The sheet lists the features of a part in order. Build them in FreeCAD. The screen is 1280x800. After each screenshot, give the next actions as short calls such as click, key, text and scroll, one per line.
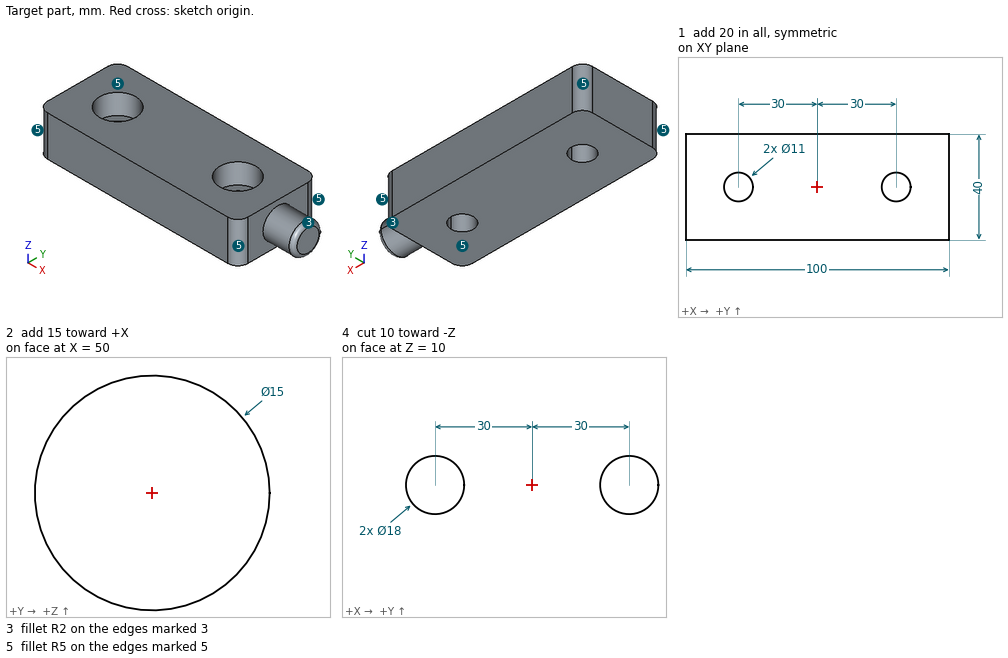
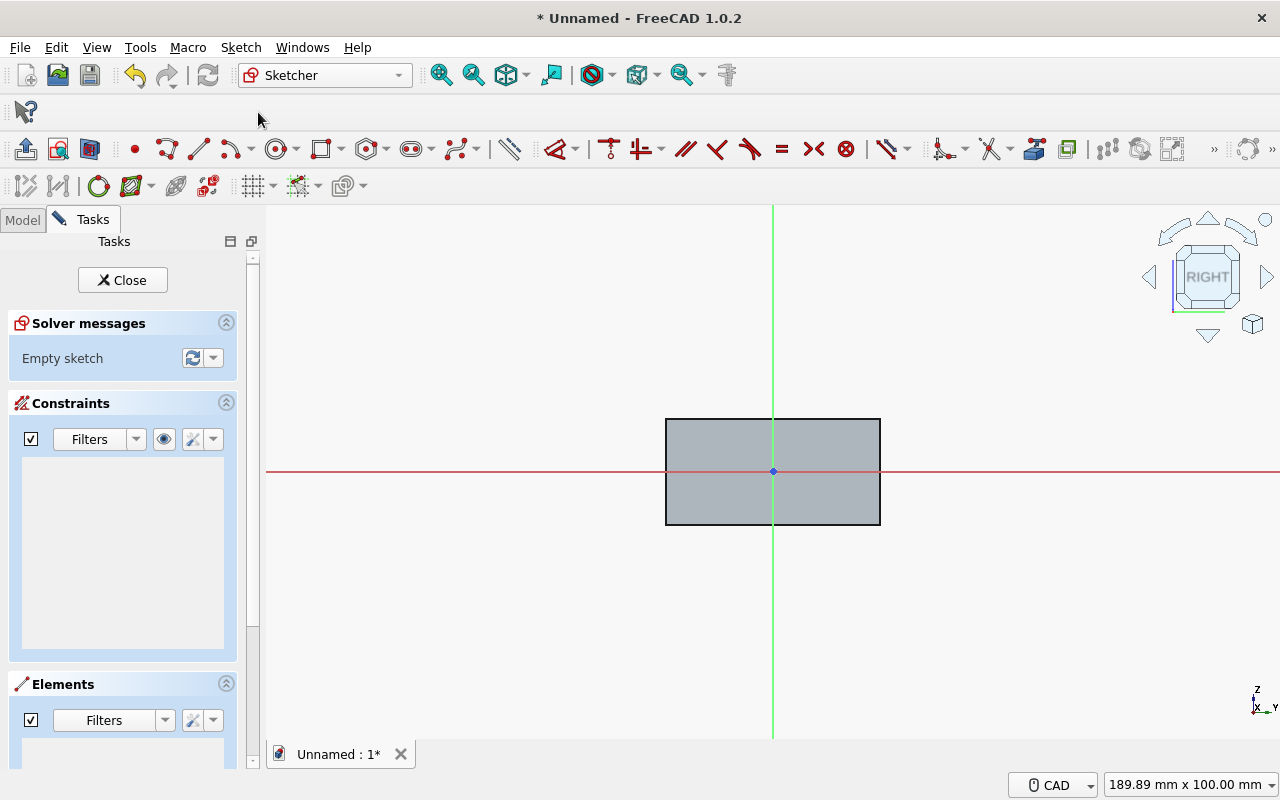
scroll(795, 472, up, 7)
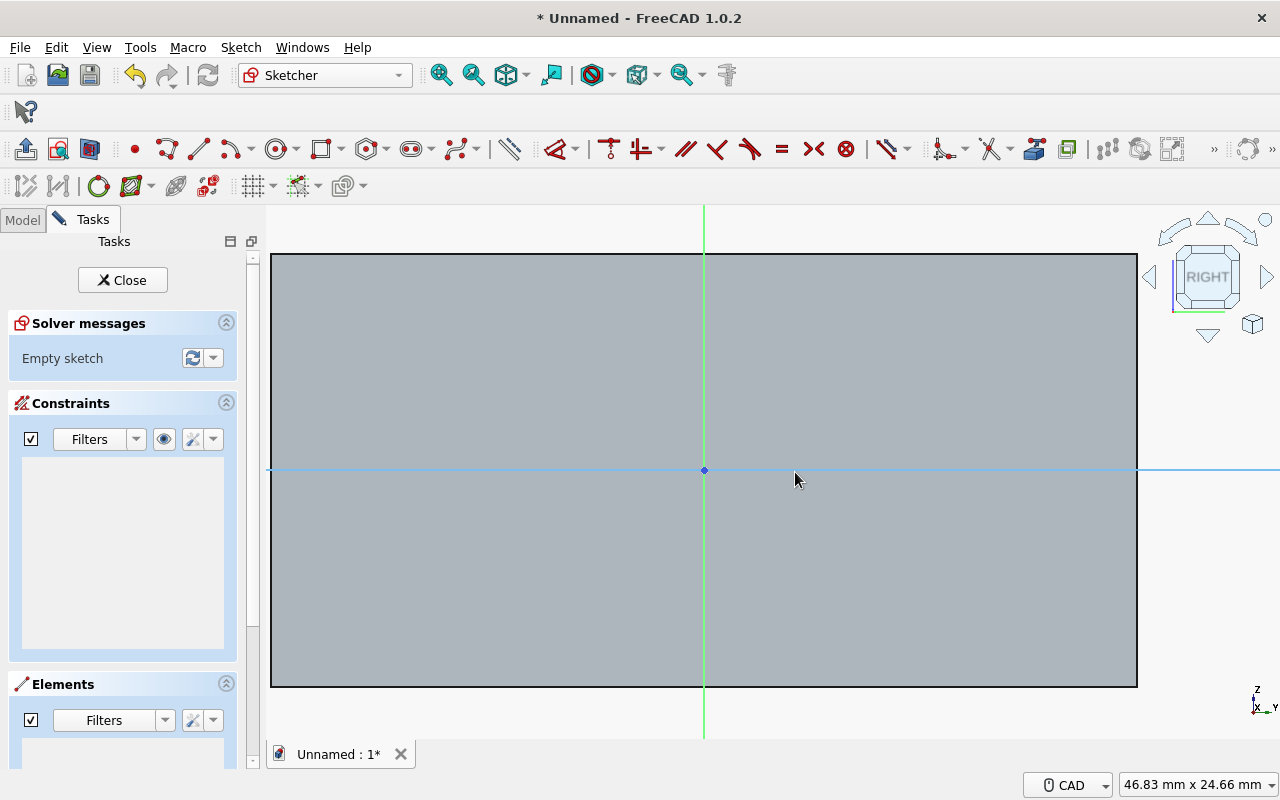
key(g)
key(c)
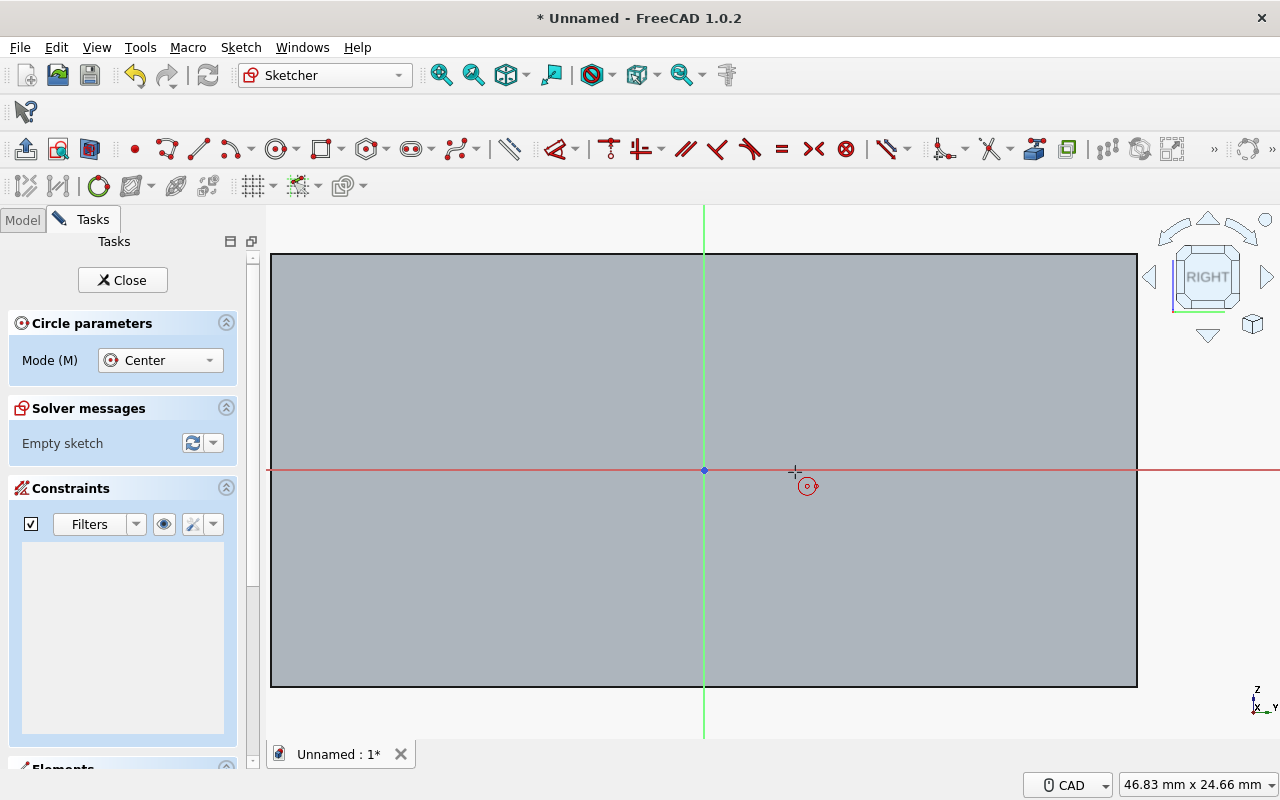
click(704, 470)
click(819, 356)
key(Escape)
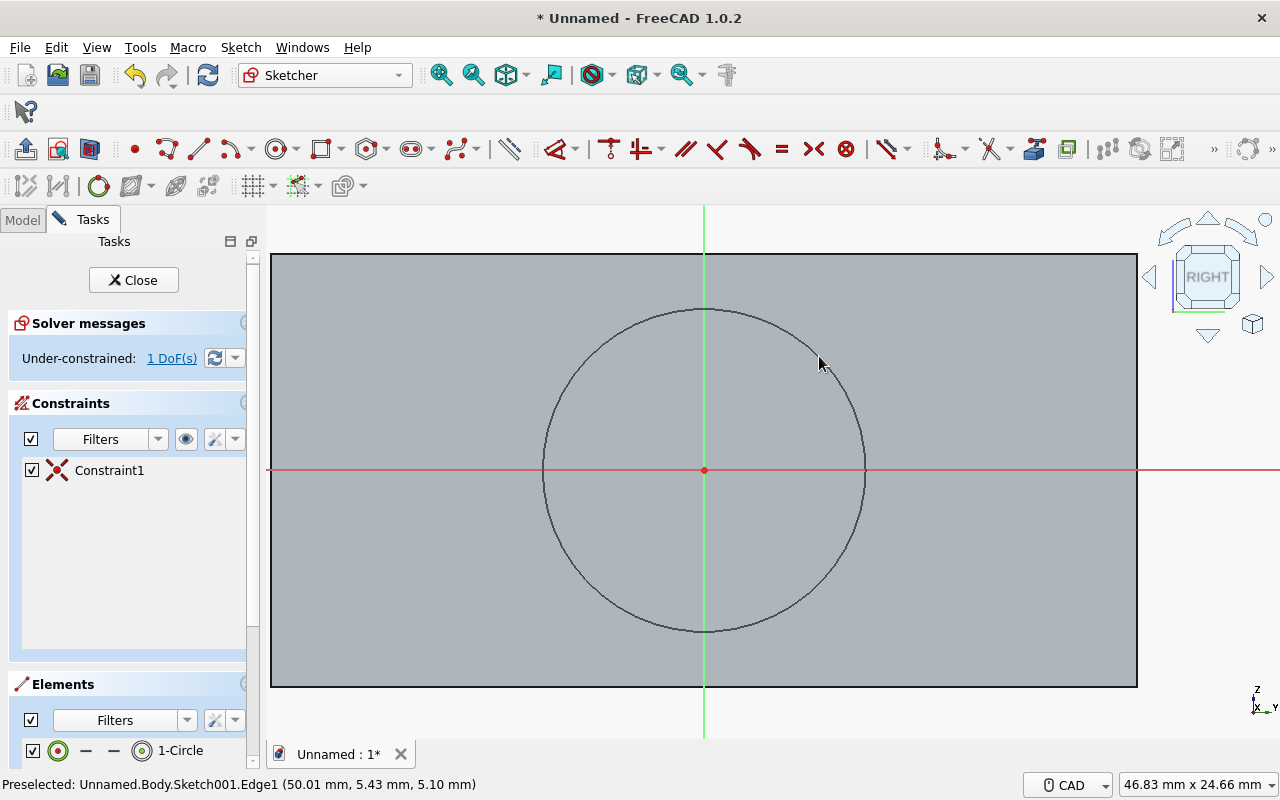
click(556, 150)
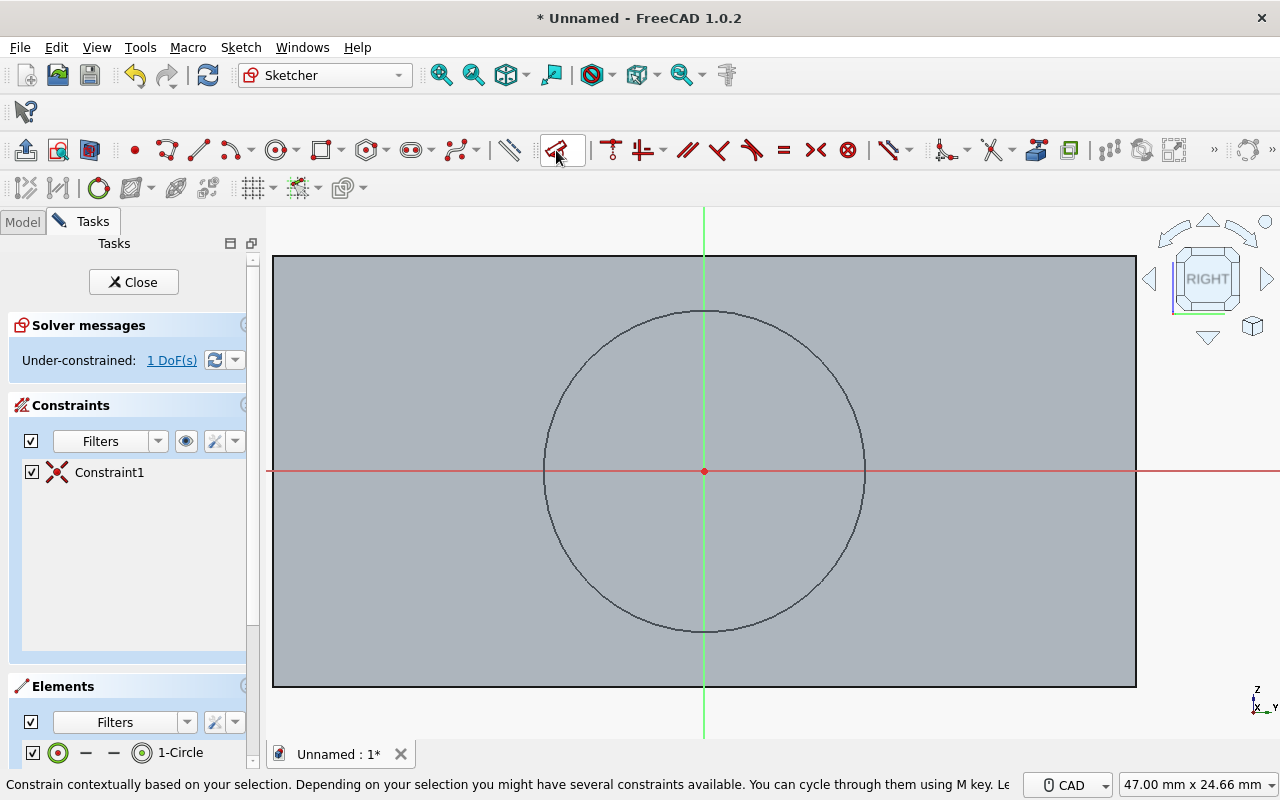
click(818, 357)
click(841, 334)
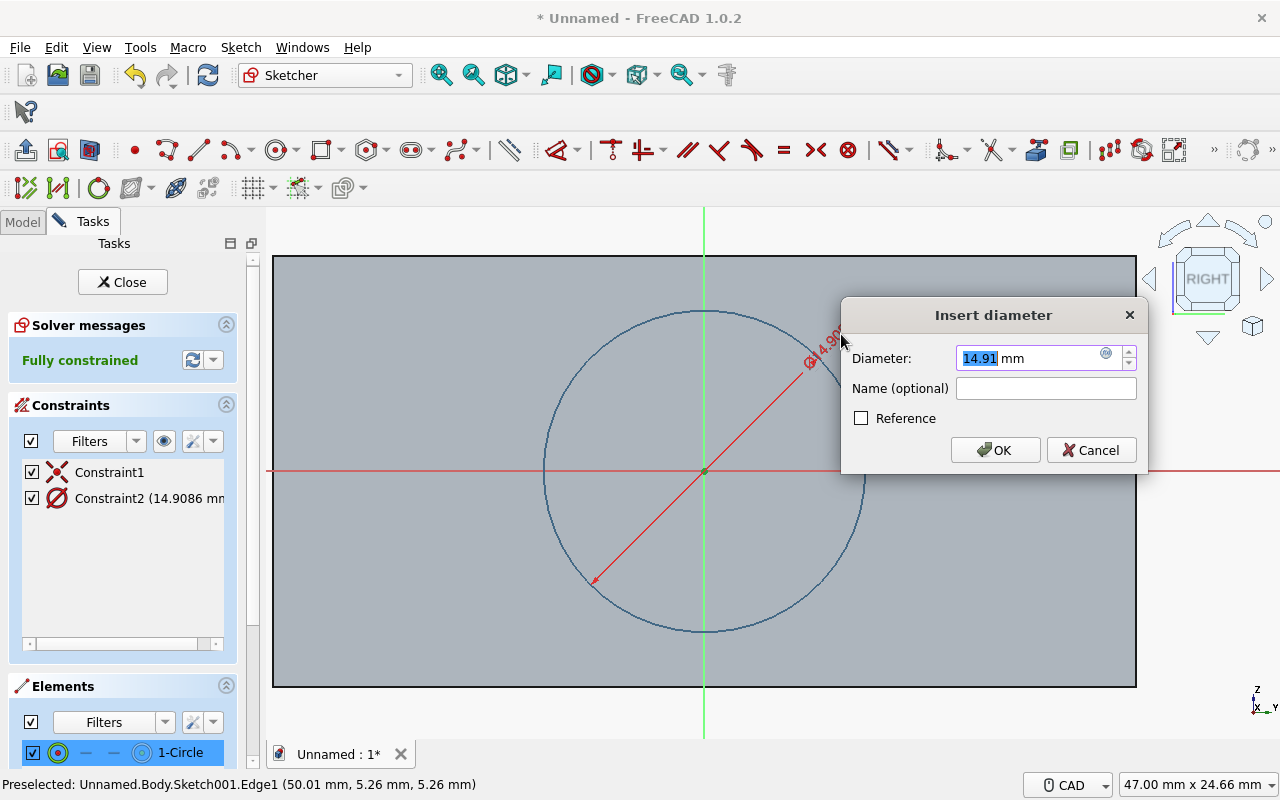
text(15)
key(Return)
key(Escape)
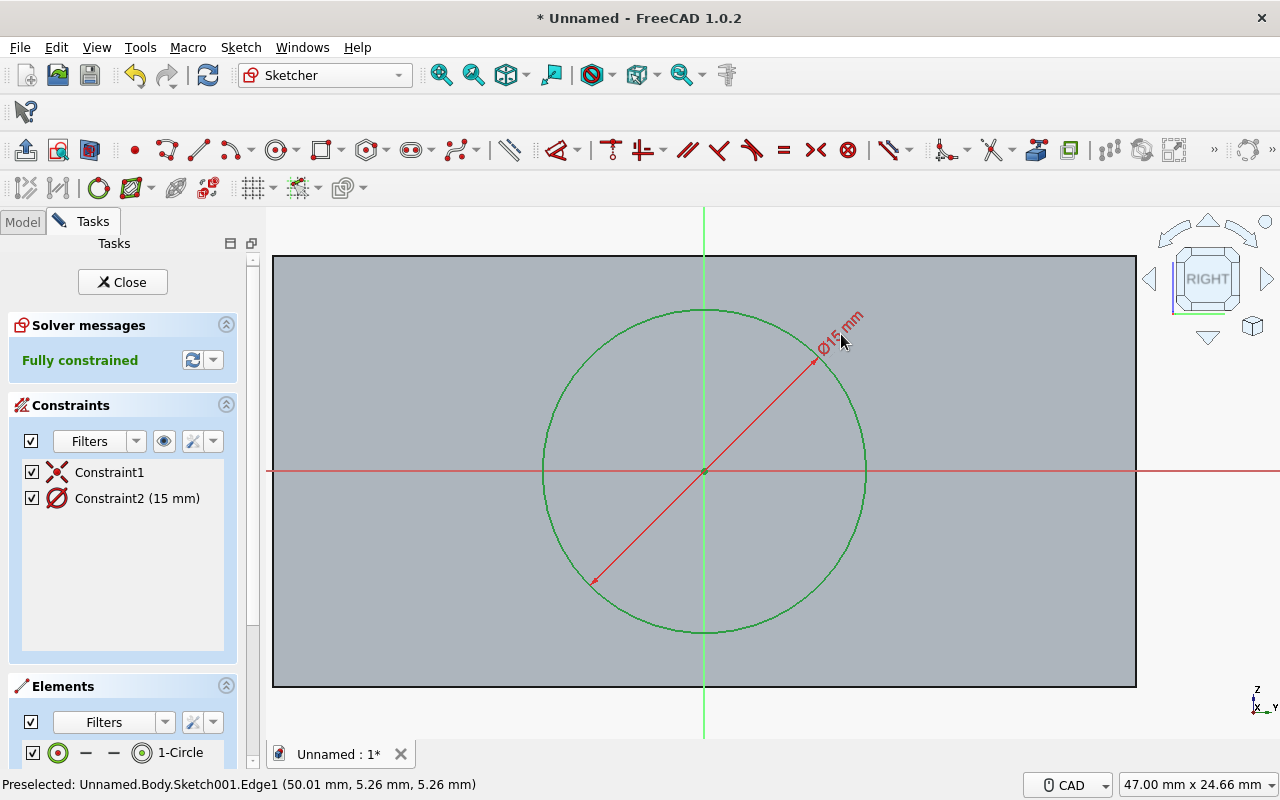
click(123, 282)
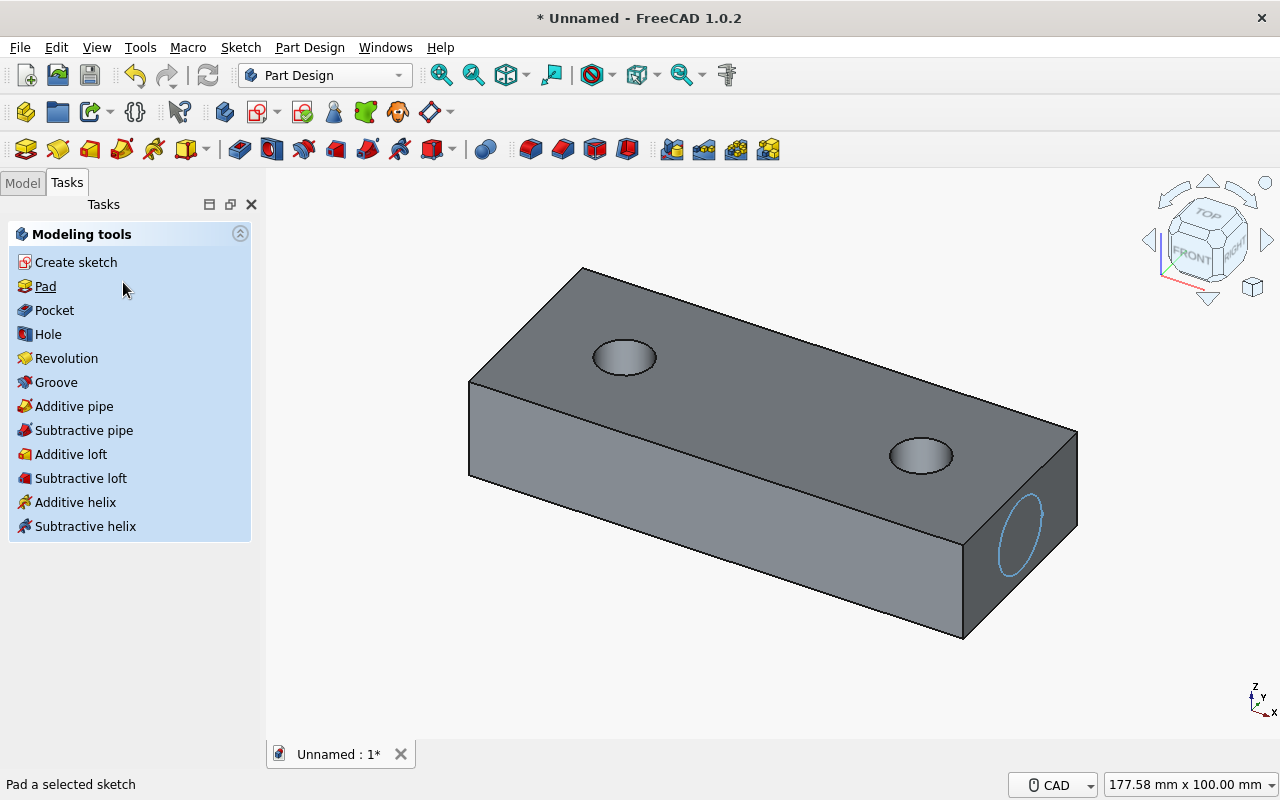
click(26, 150)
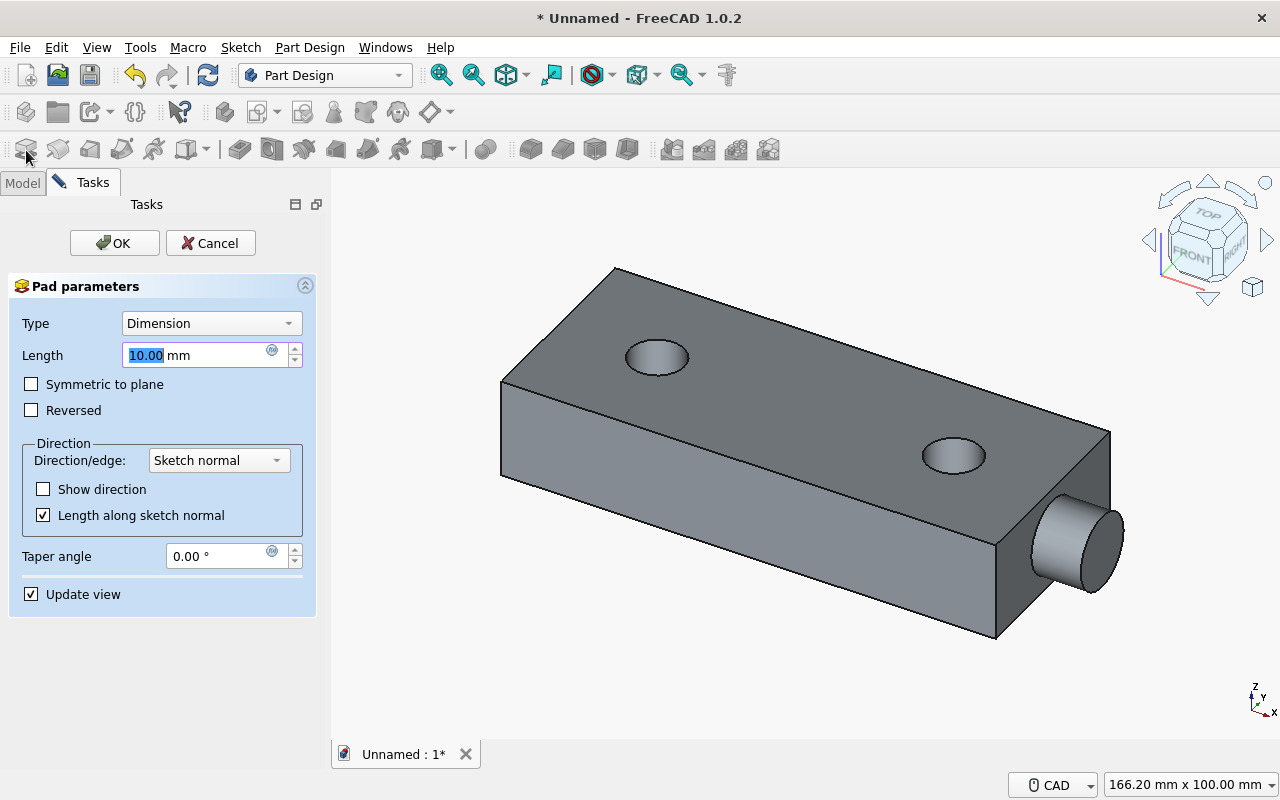
text(15)
key(Tab)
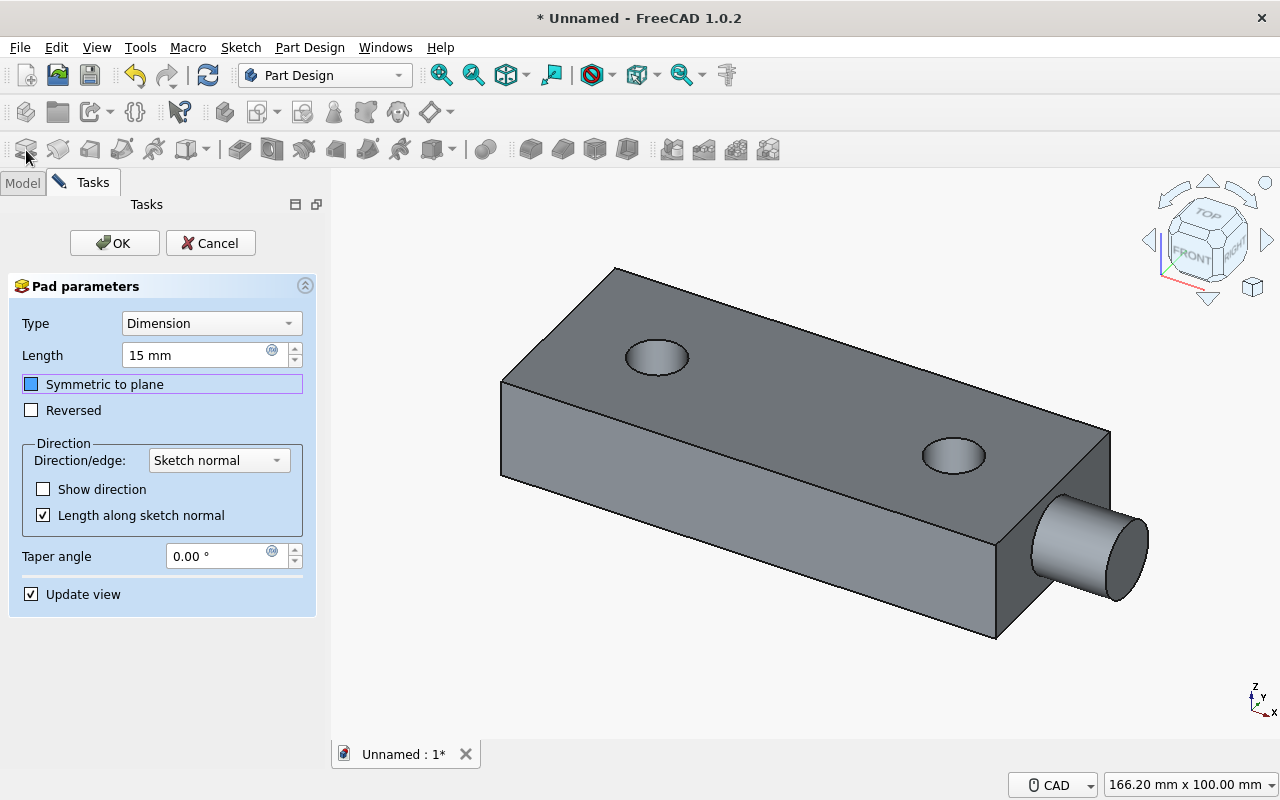
click(115, 243)